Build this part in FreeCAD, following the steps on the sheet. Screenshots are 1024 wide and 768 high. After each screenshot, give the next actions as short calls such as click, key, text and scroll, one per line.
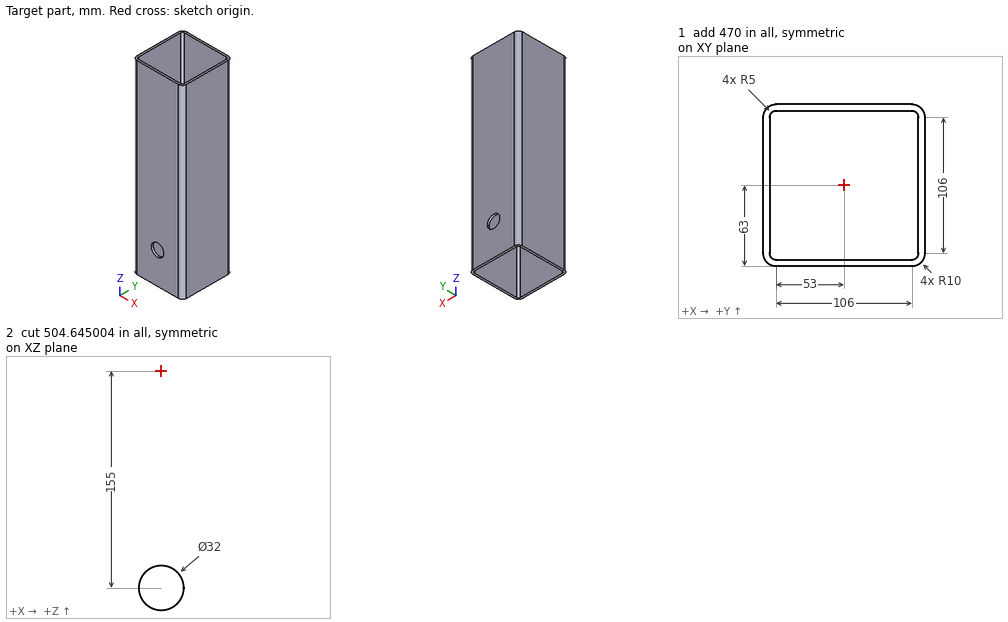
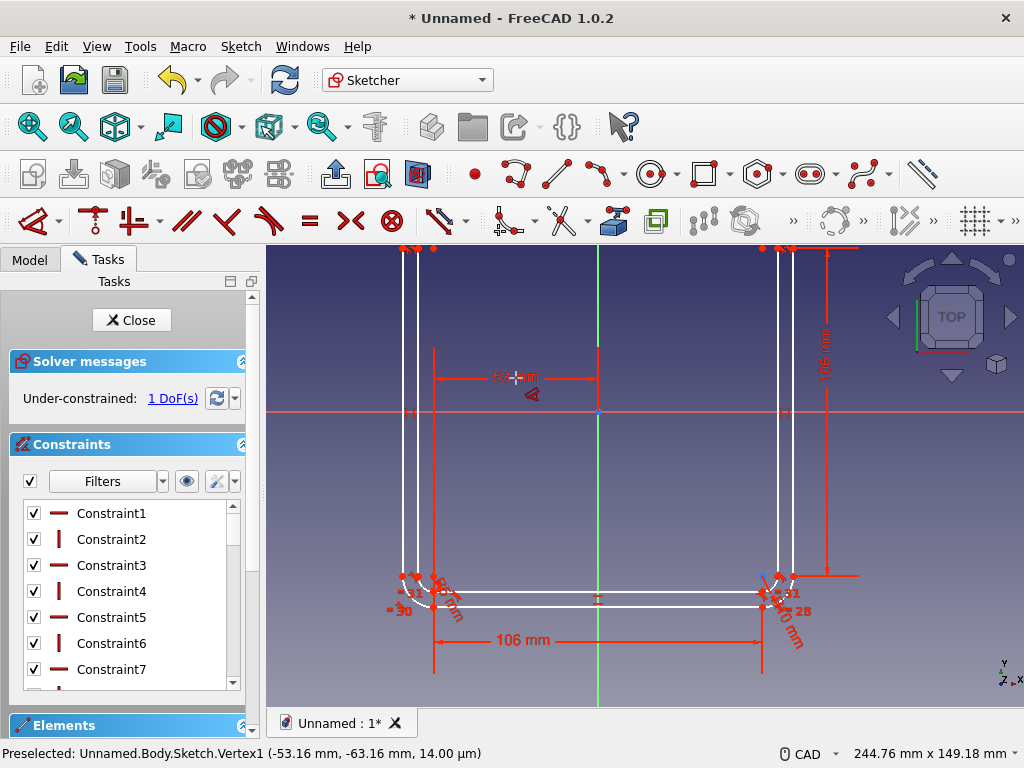
click(434, 607)
click(632, 510)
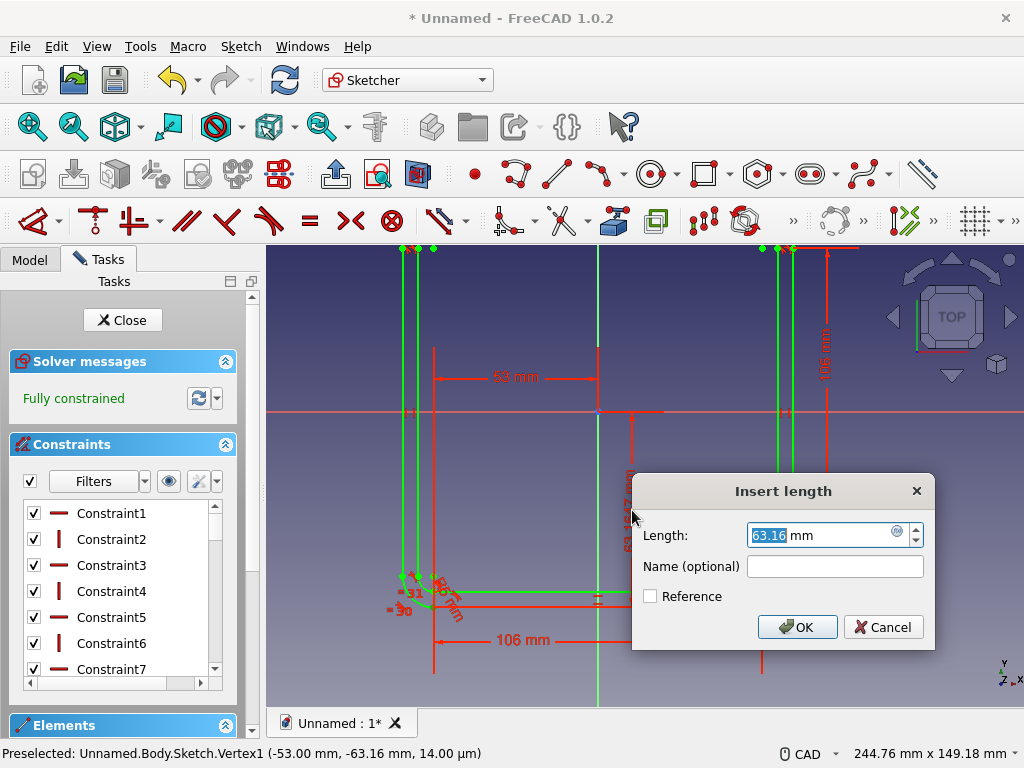
text(63)
key(Return)
key(Escape)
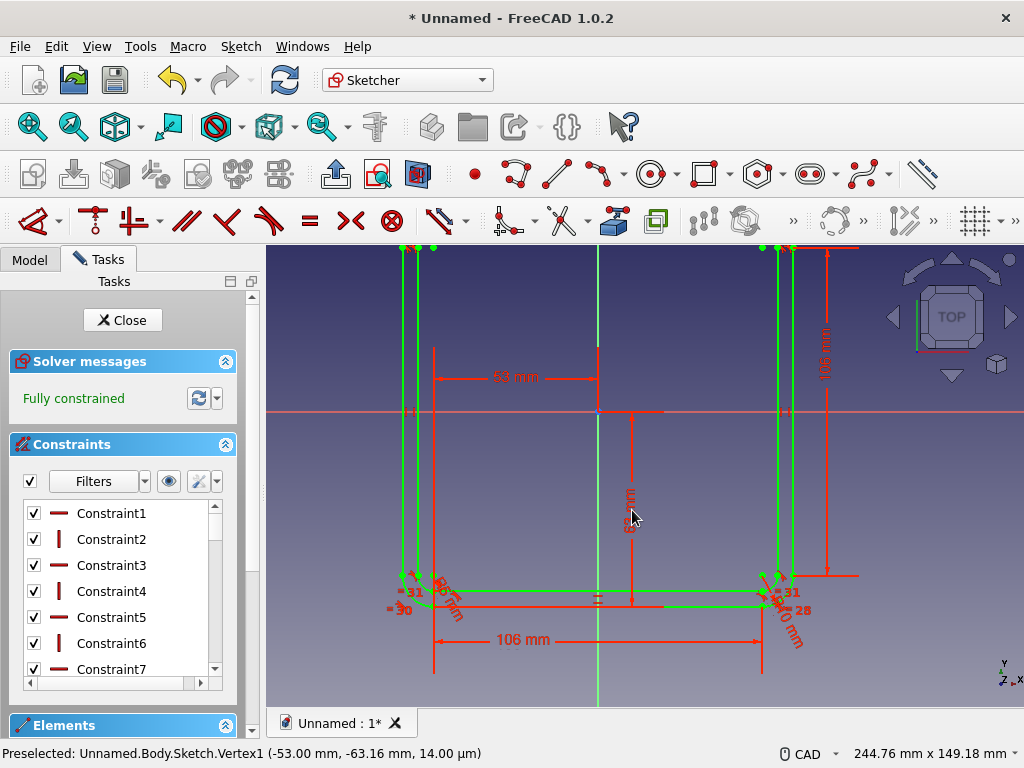
click(123, 320)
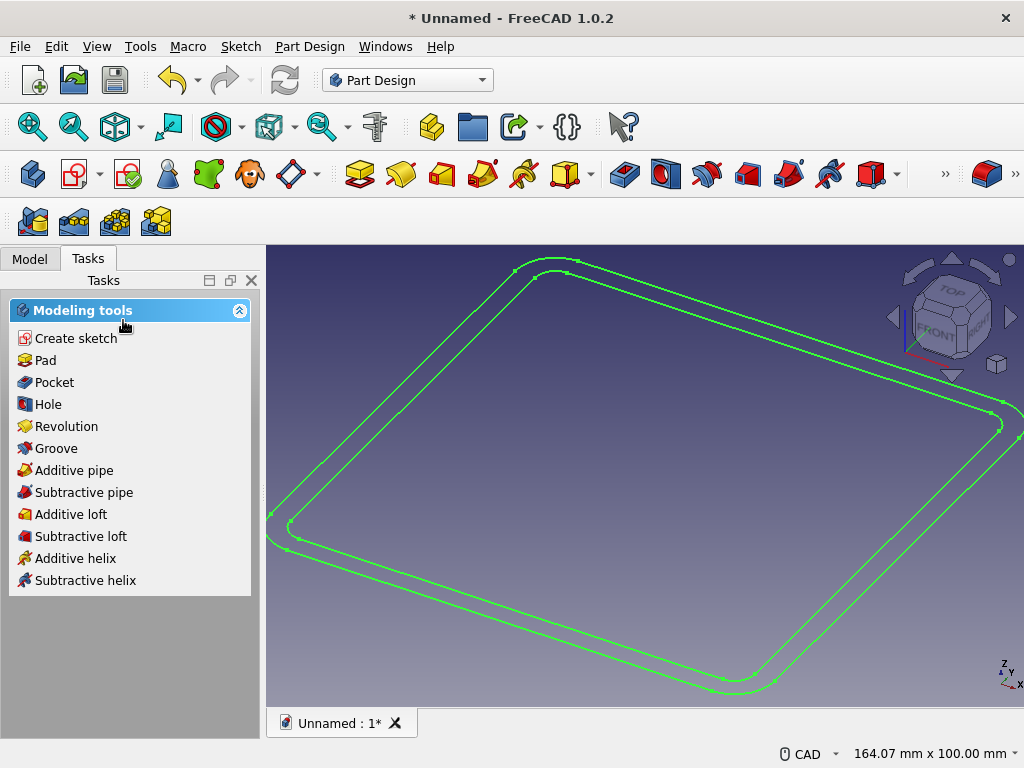
click(360, 174)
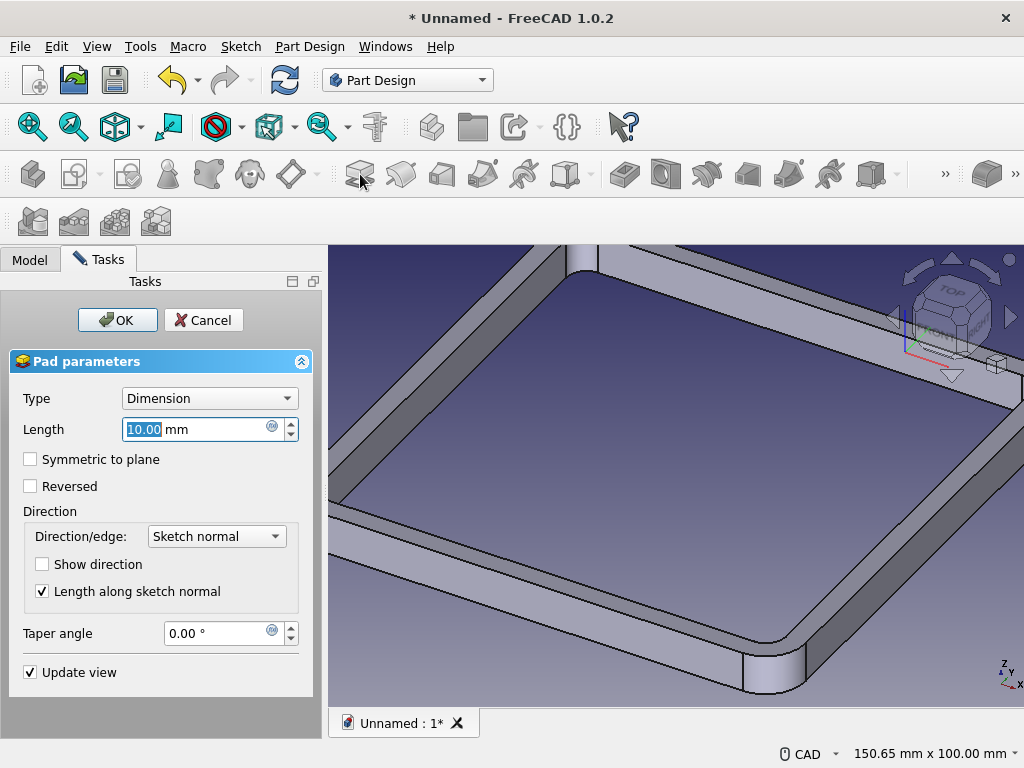
text(470)
key(Tab)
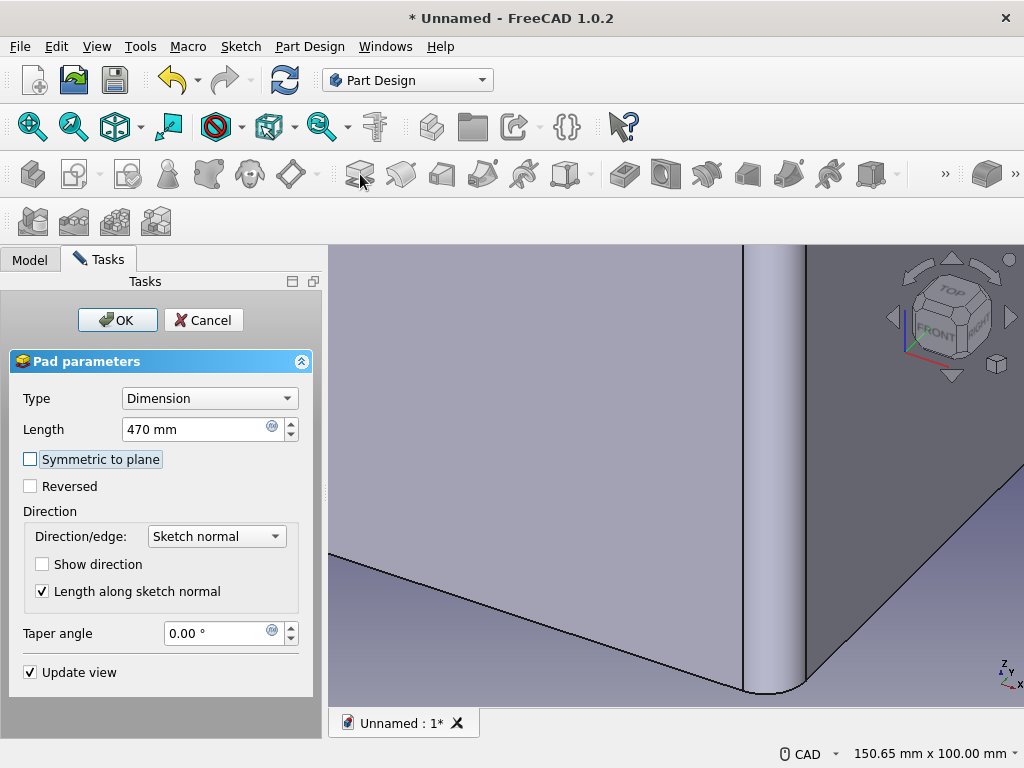
click(31, 459)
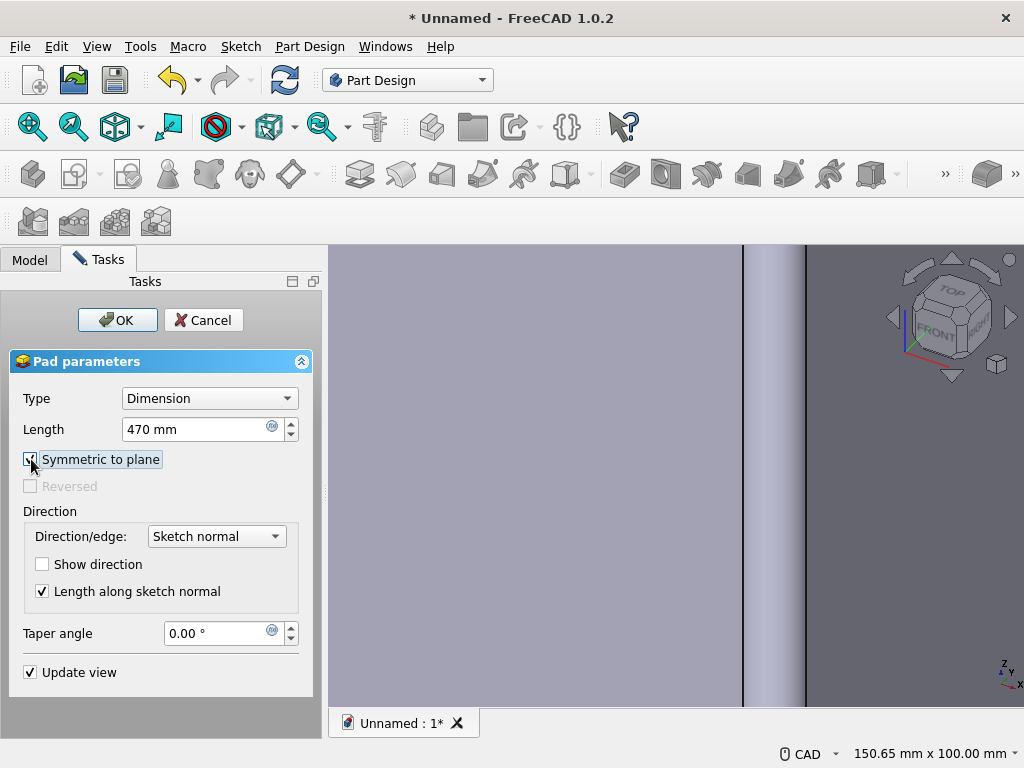
click(118, 320)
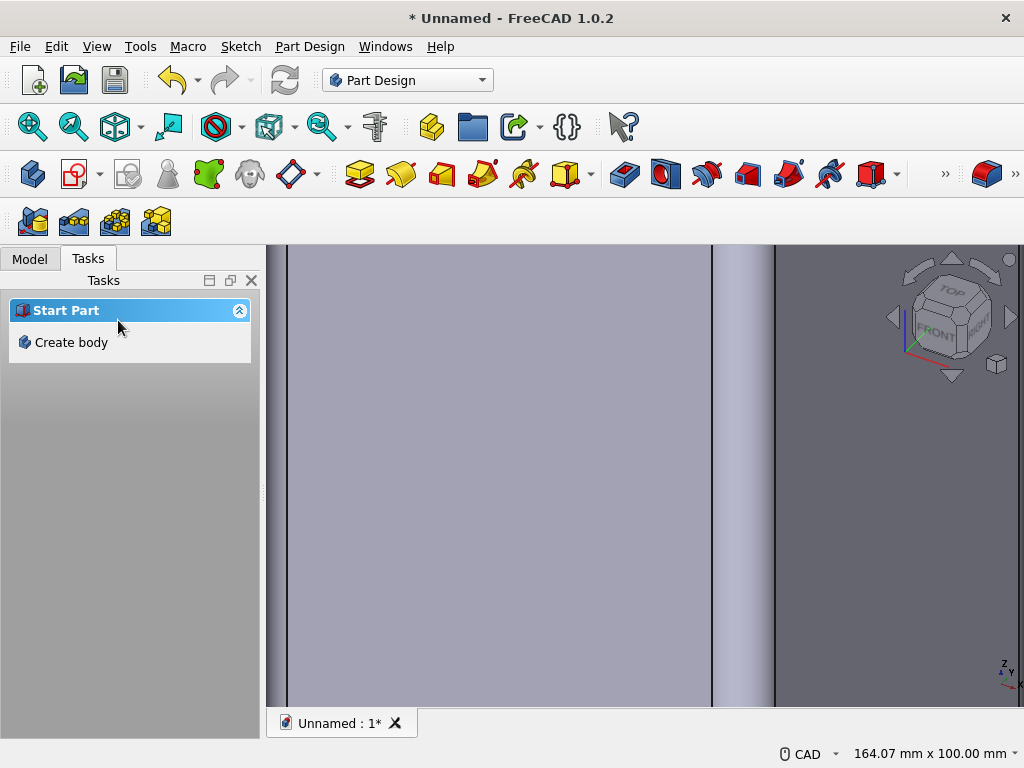
click(33, 128)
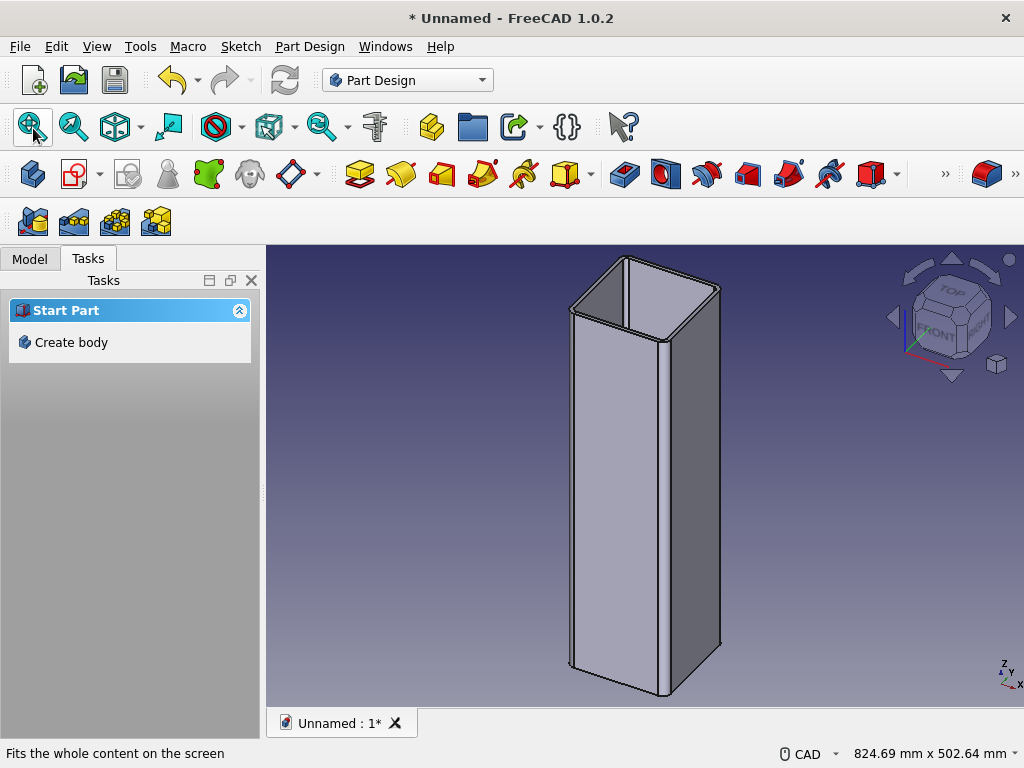
click(74, 174)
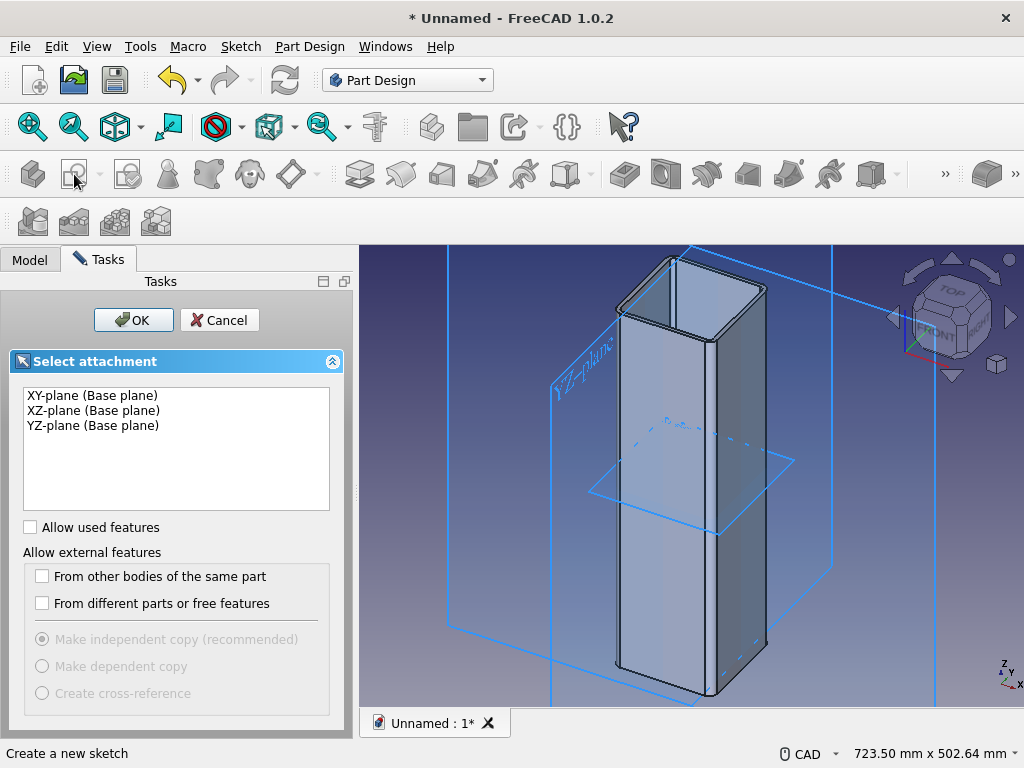
click(84, 410)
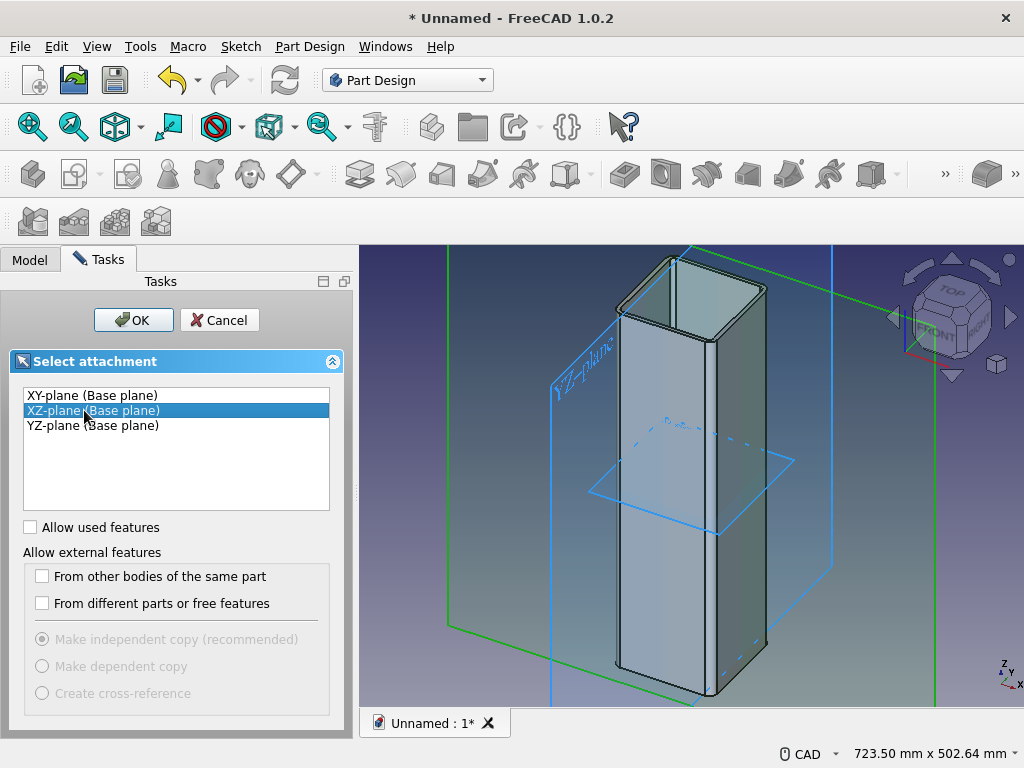
click(134, 320)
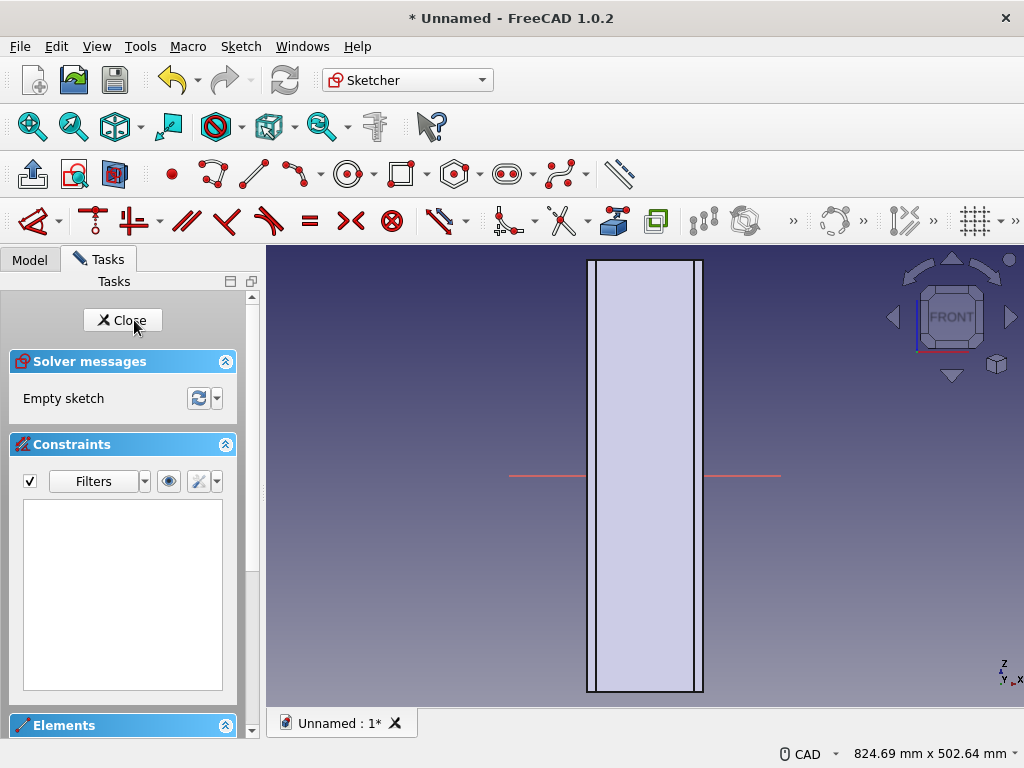
key(q)
key(s)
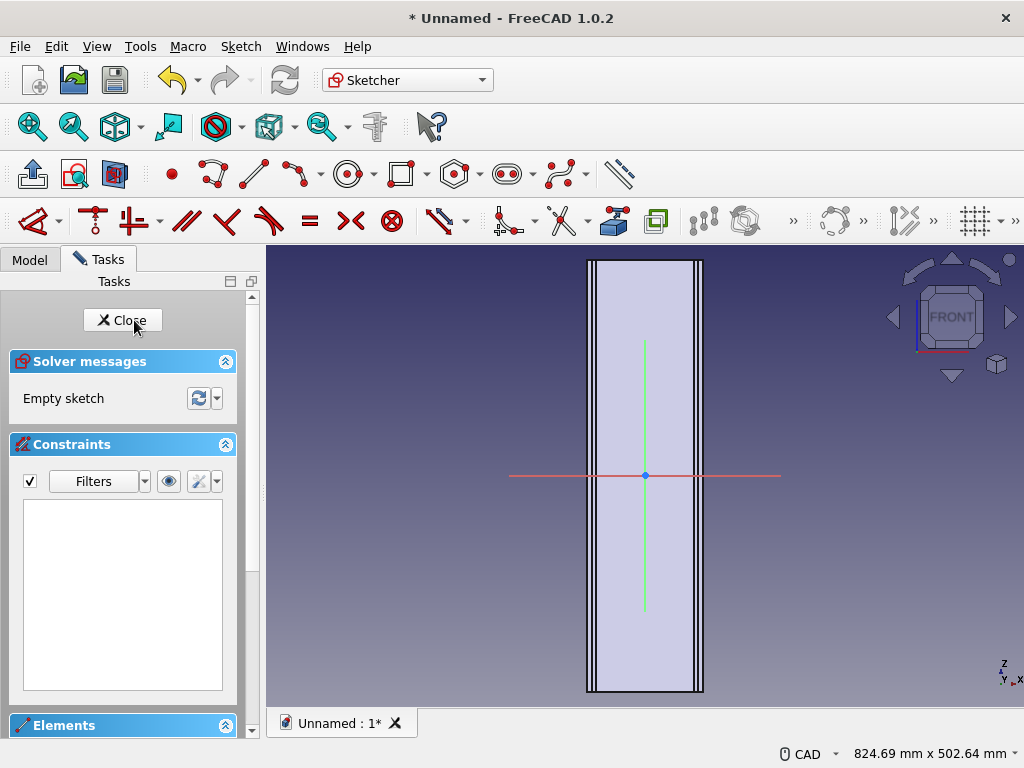
scroll(654, 636, up, 11)